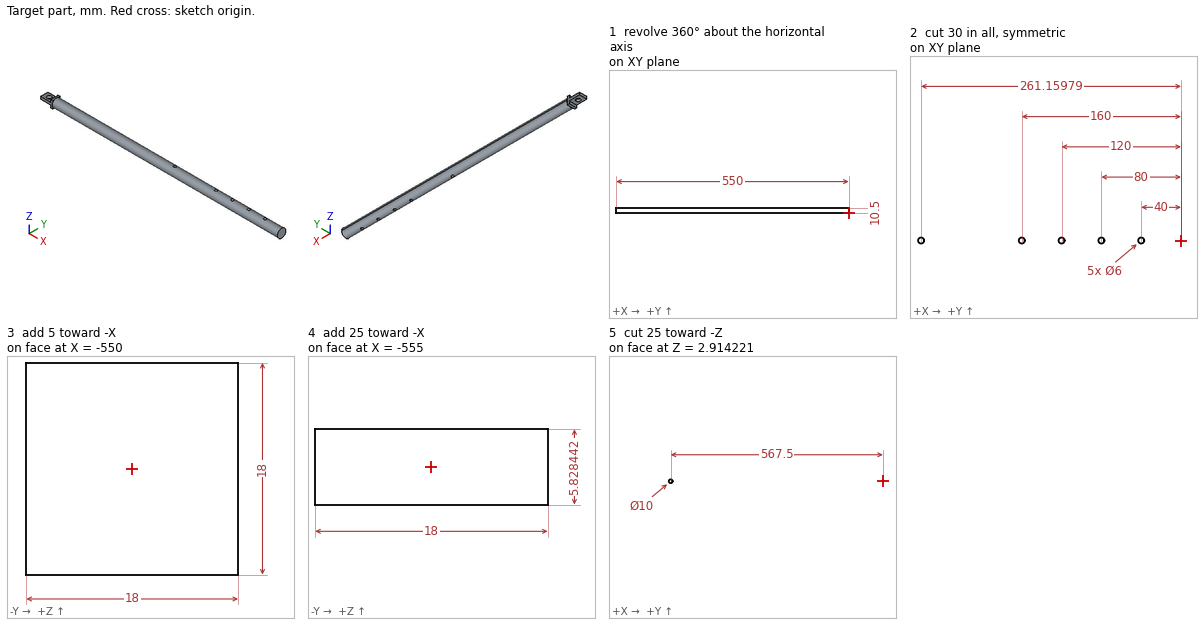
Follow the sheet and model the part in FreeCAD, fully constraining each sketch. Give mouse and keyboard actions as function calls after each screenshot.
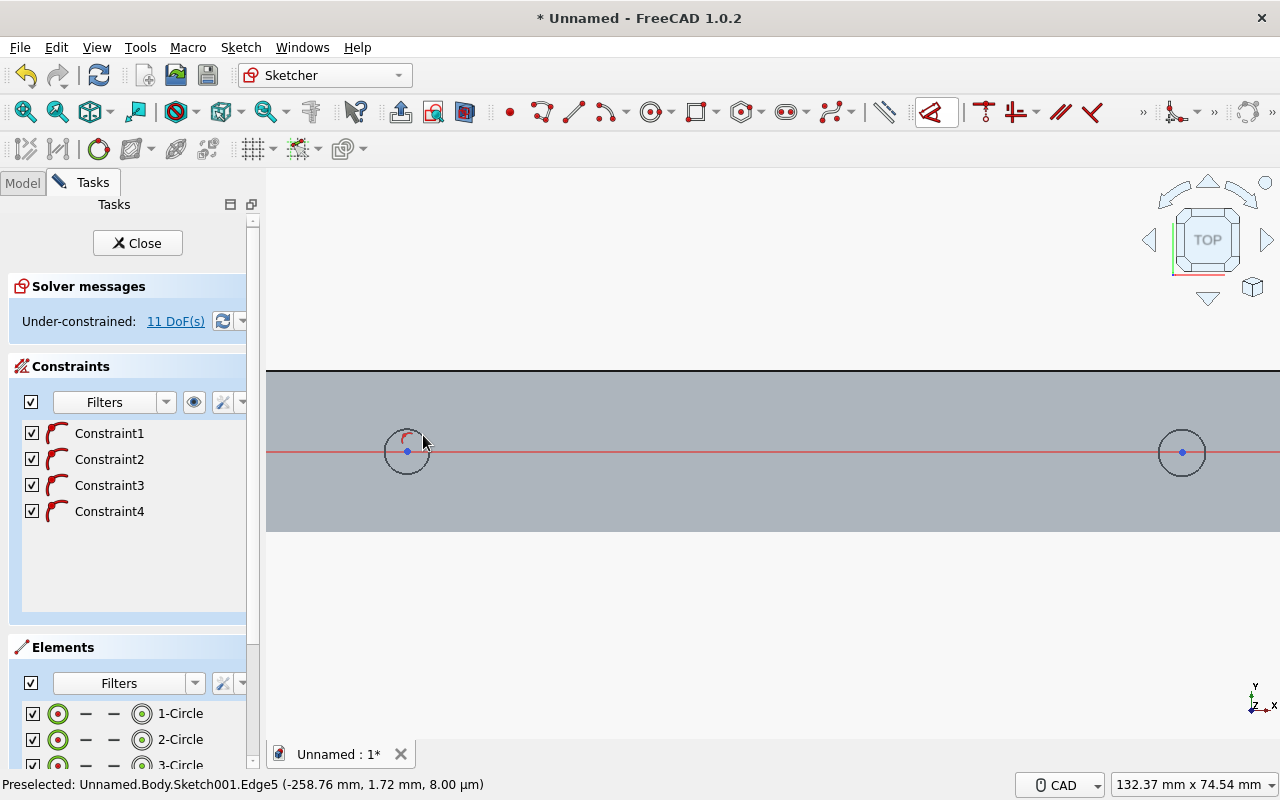
scroll(407, 454, down, 6)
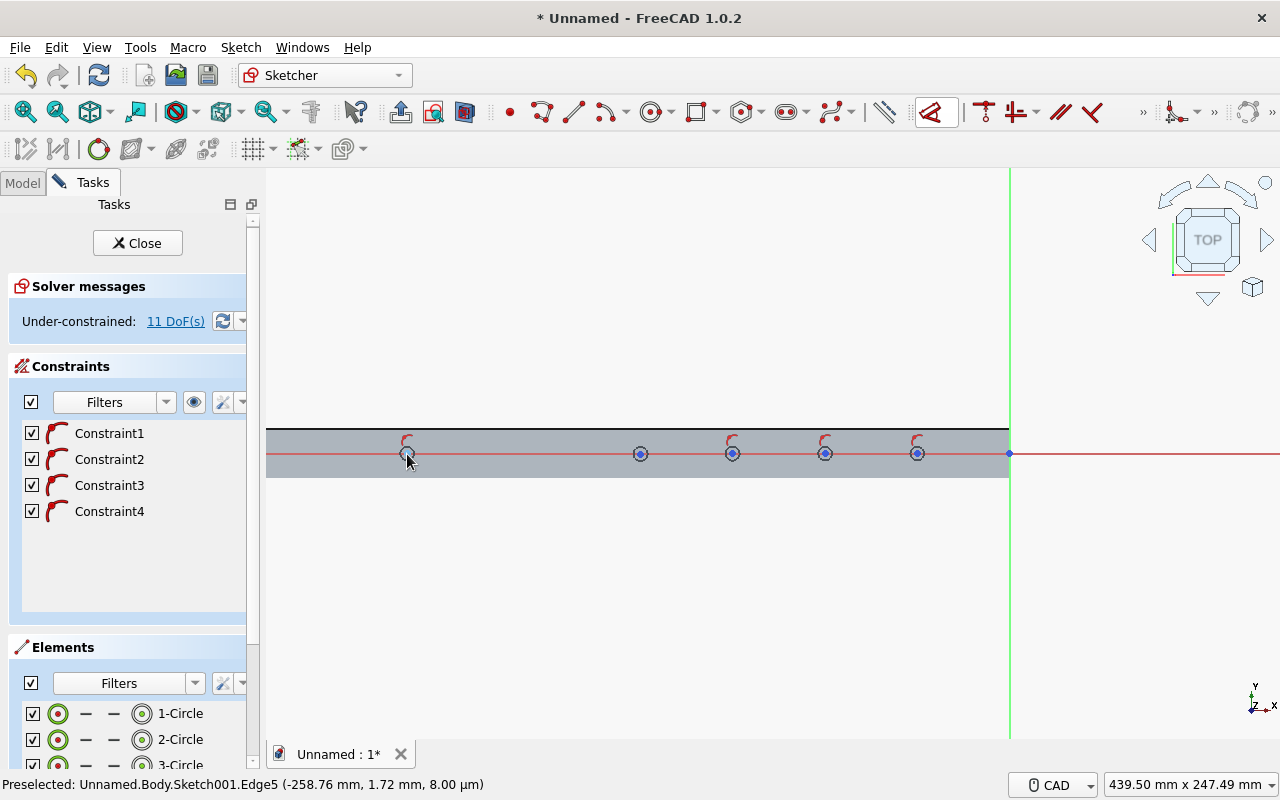
scroll(922, 449, up, 6)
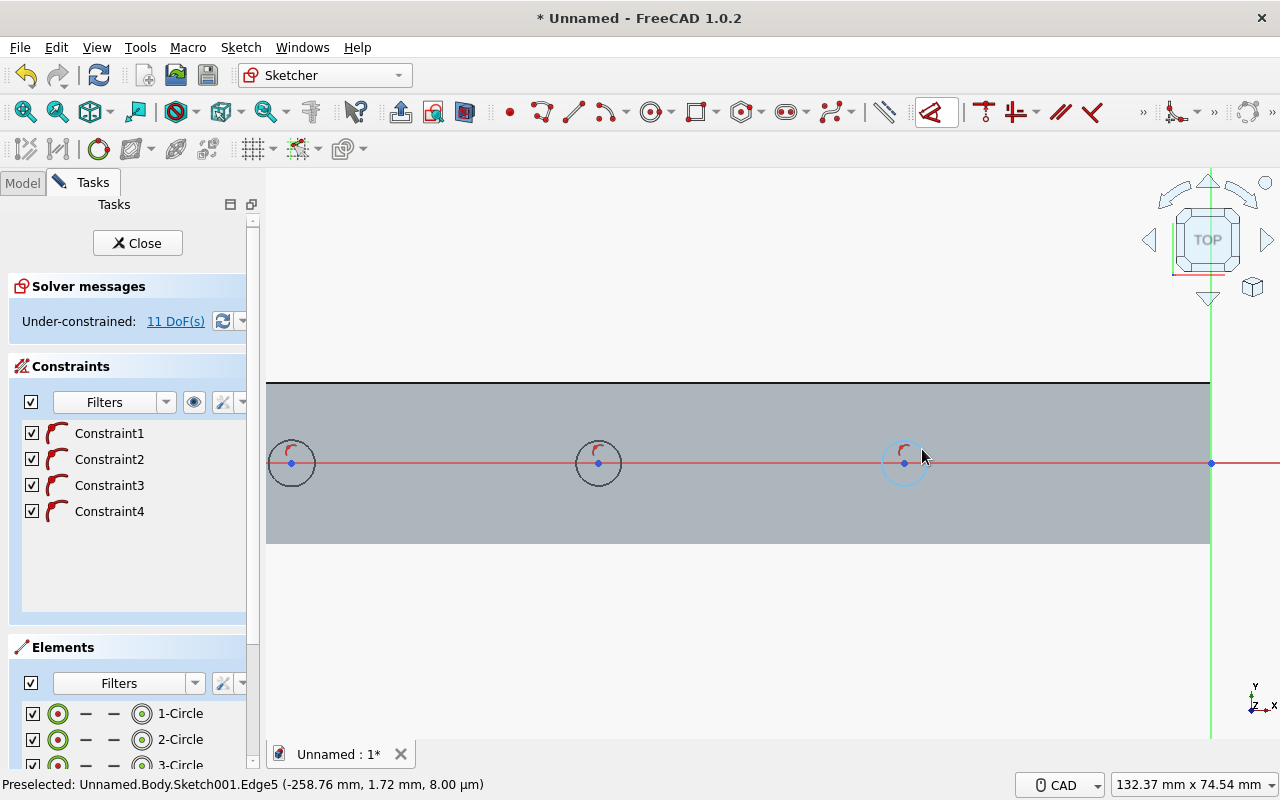
click(921, 447)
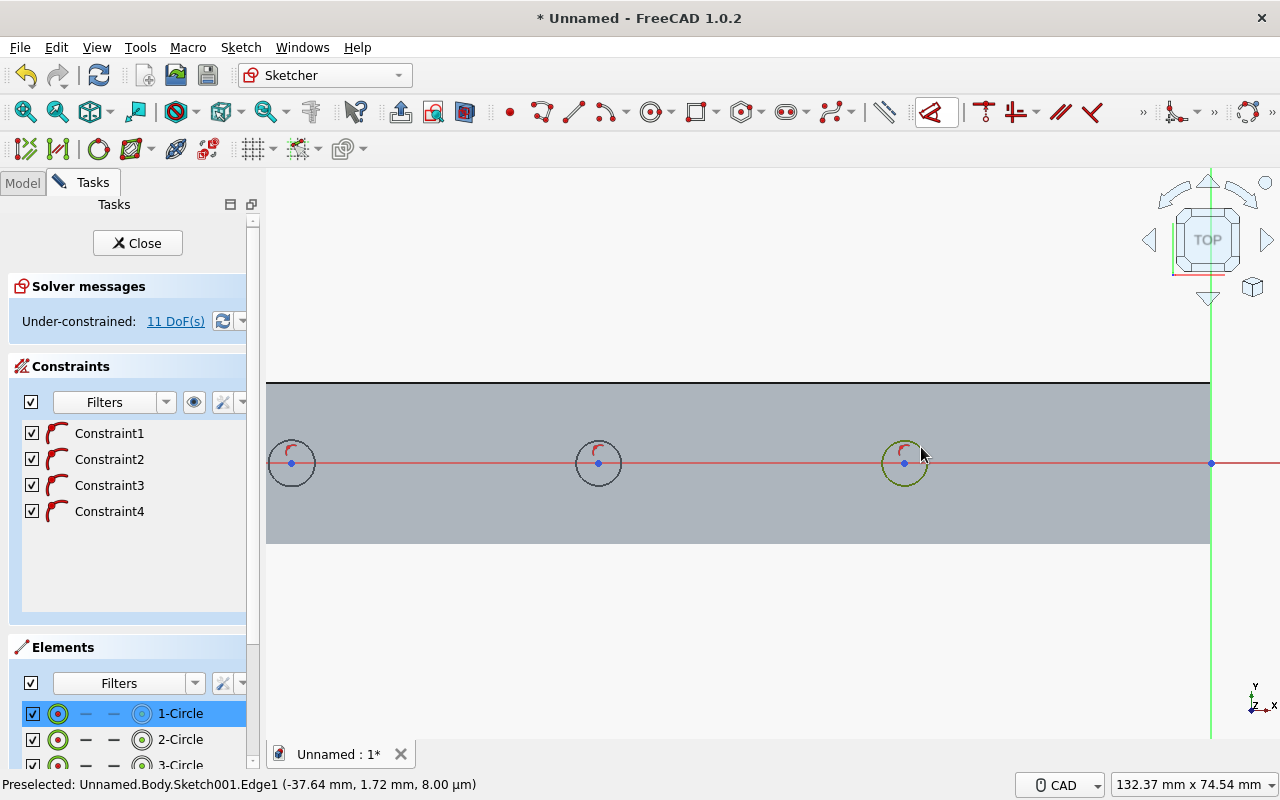
click(615, 447)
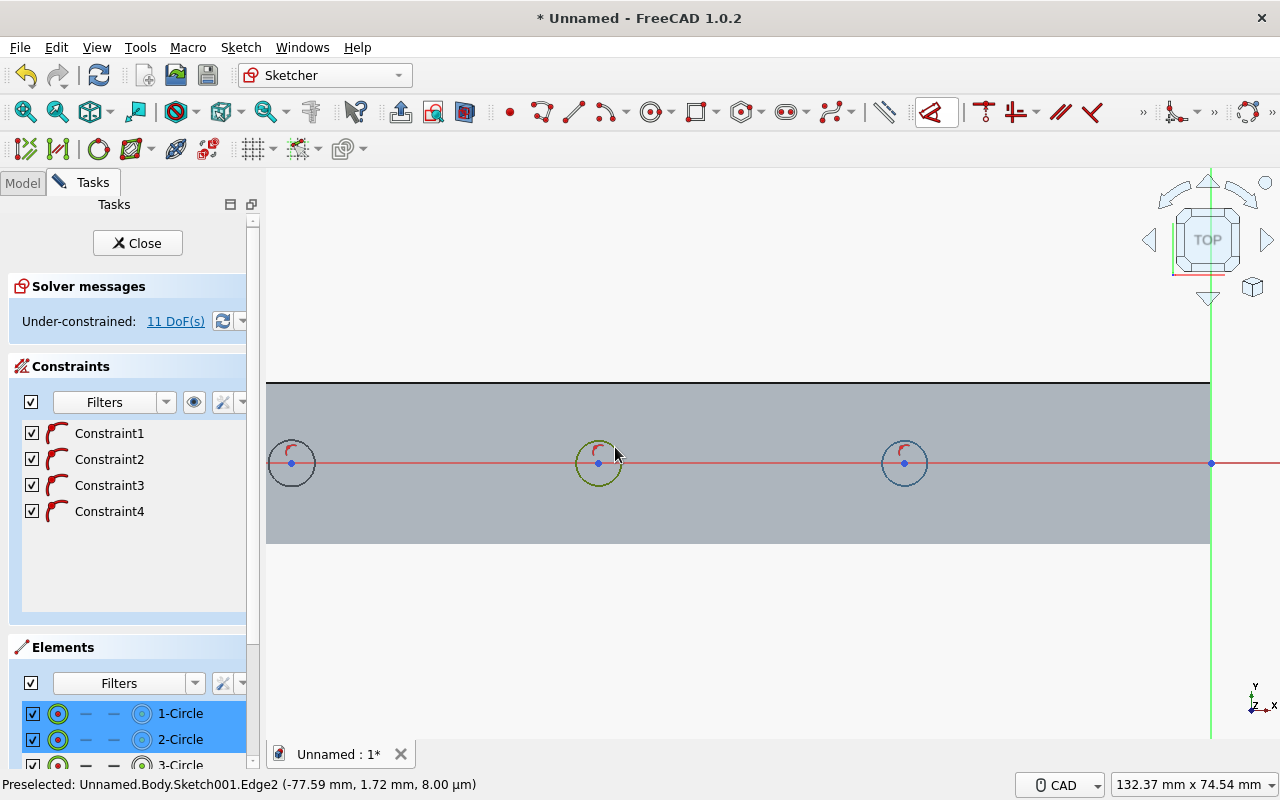
click(308, 447)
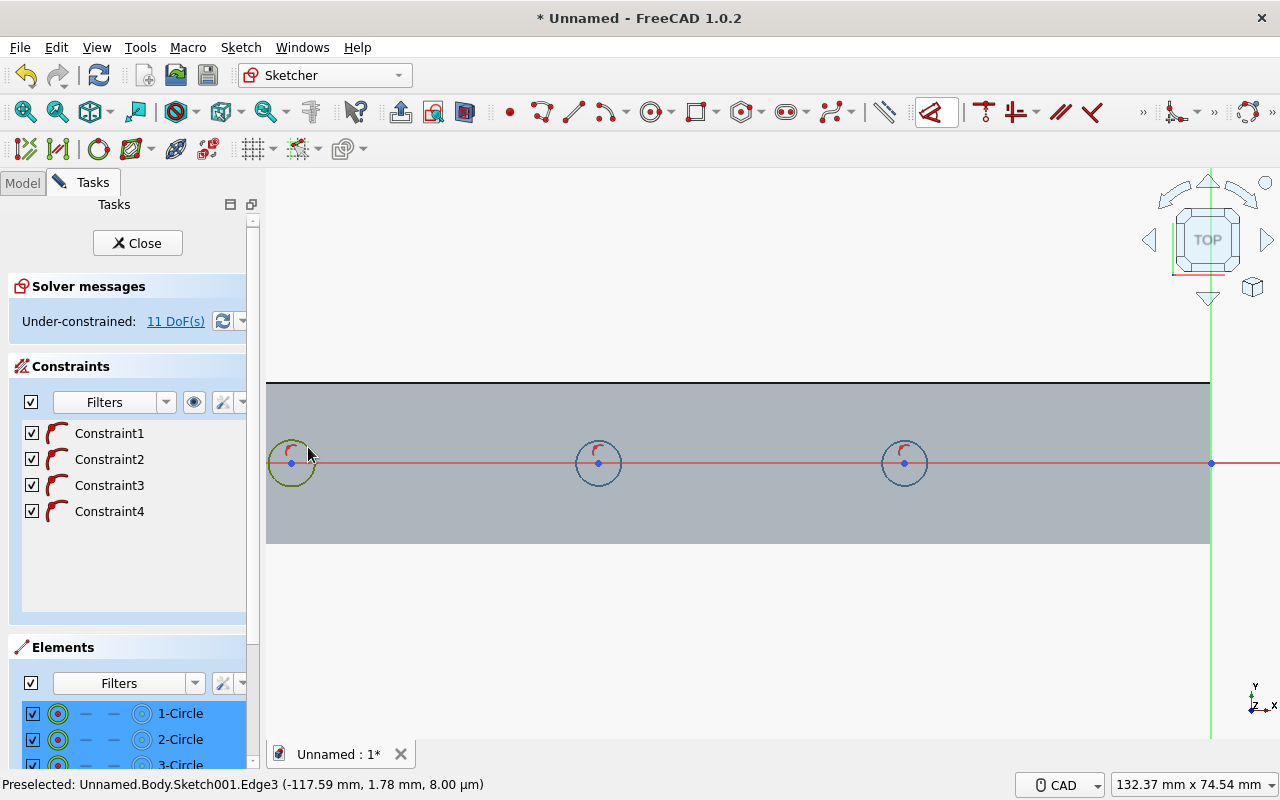
scroll(922, 449, down, 6)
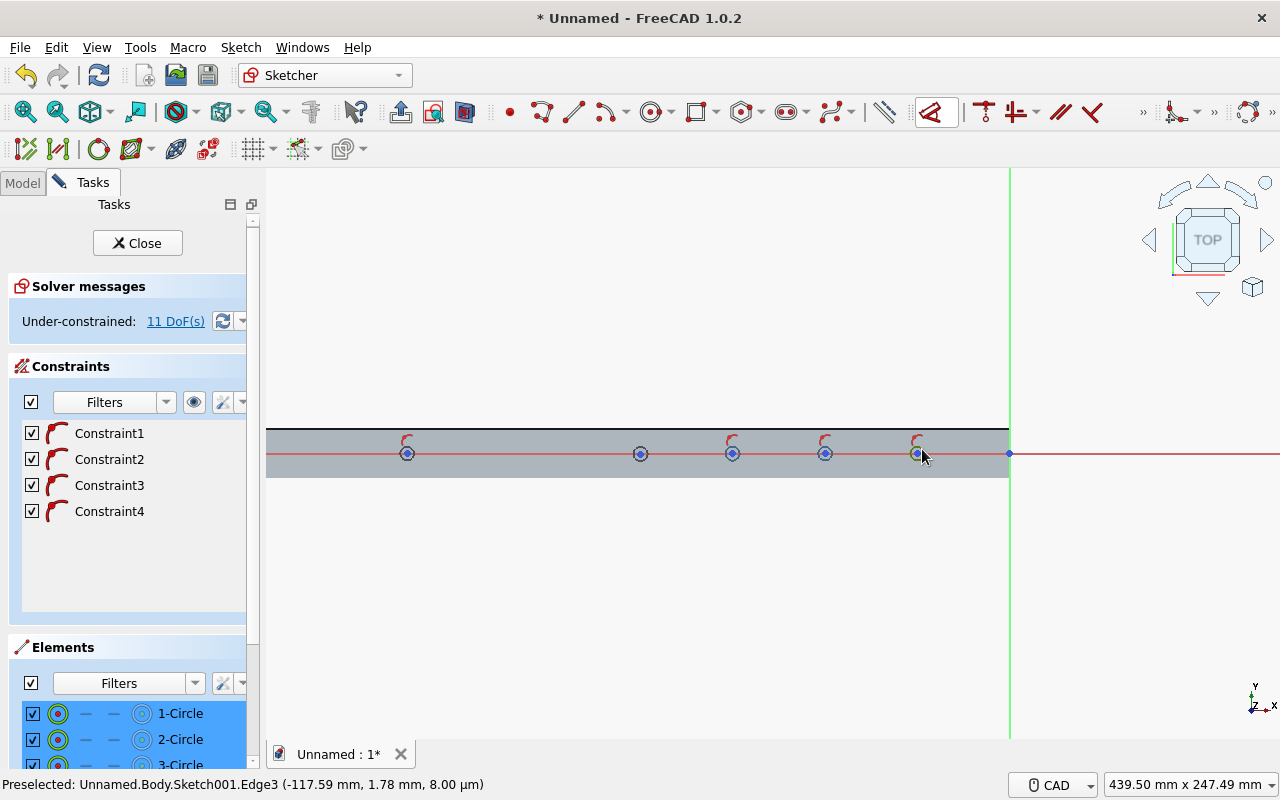
scroll(646, 449, up, 6)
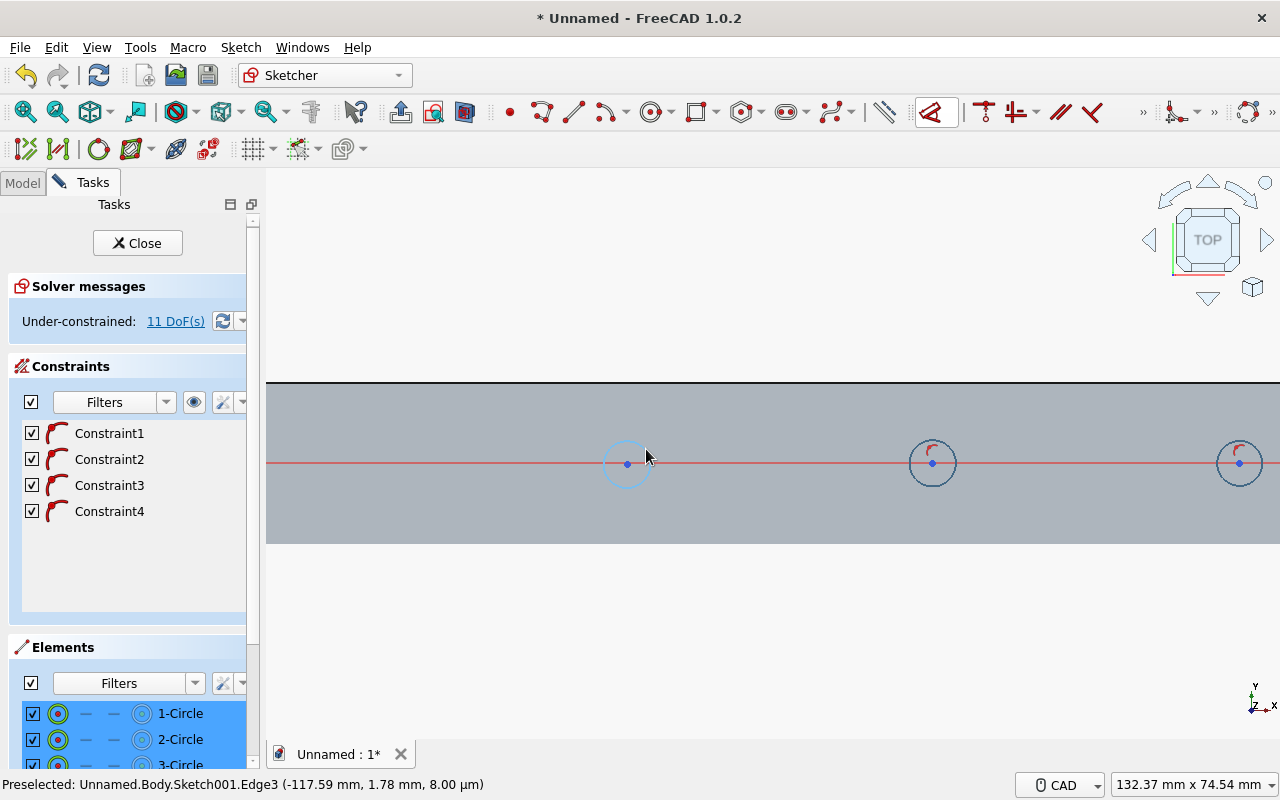
click(644, 448)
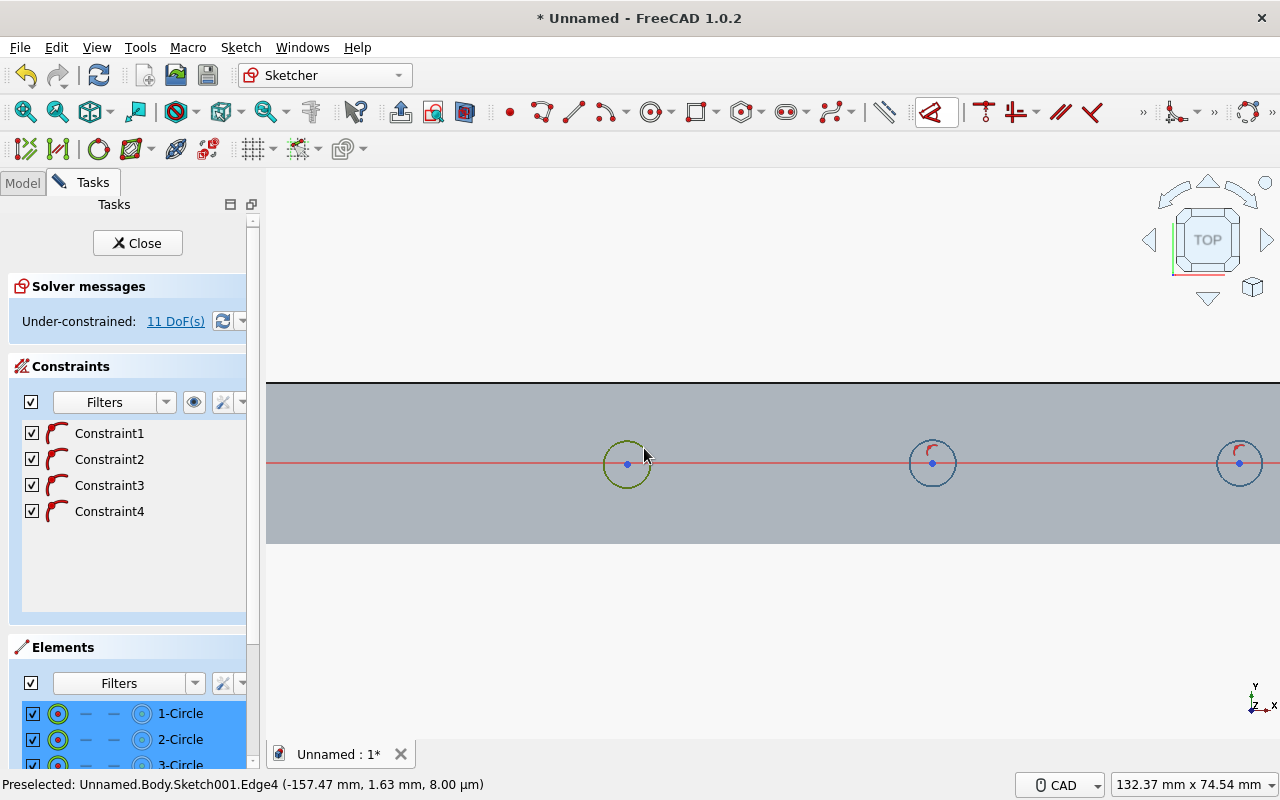
scroll(646, 449, down, 6)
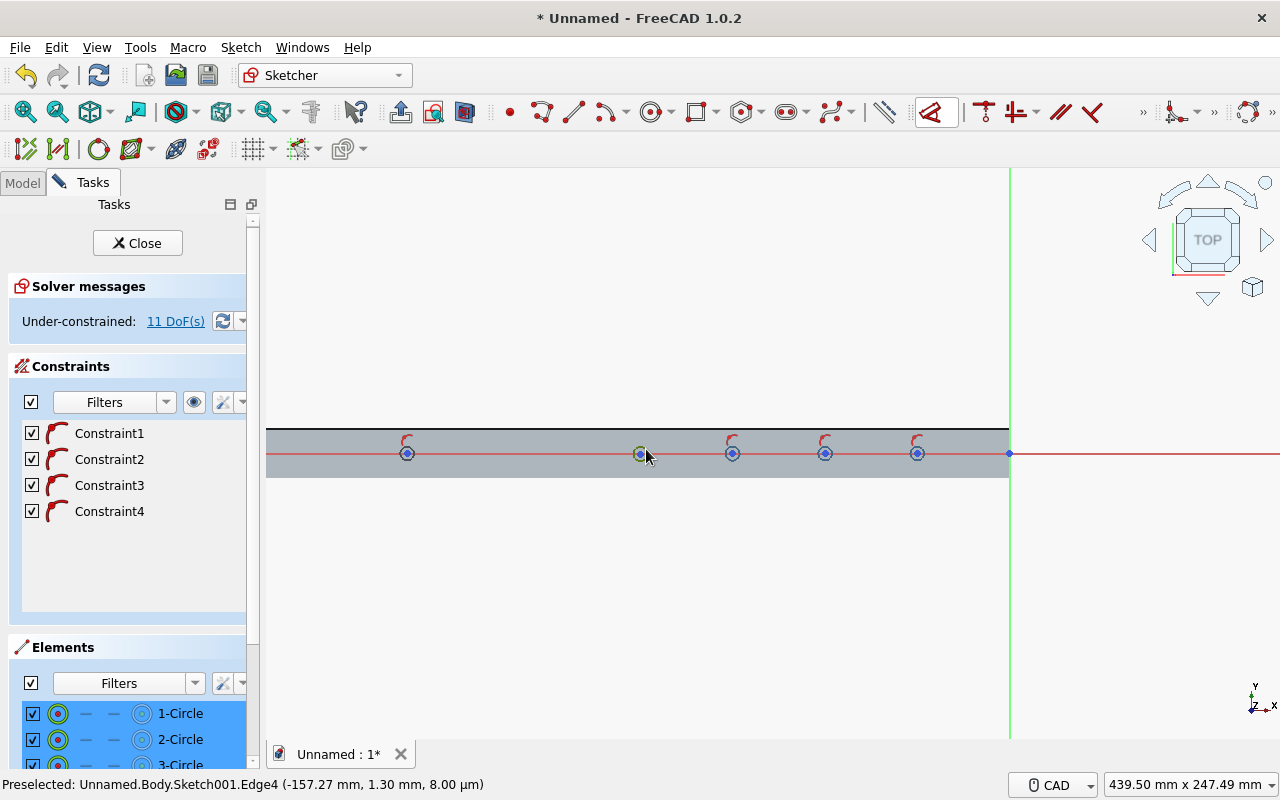
scroll(412, 449, up, 6)